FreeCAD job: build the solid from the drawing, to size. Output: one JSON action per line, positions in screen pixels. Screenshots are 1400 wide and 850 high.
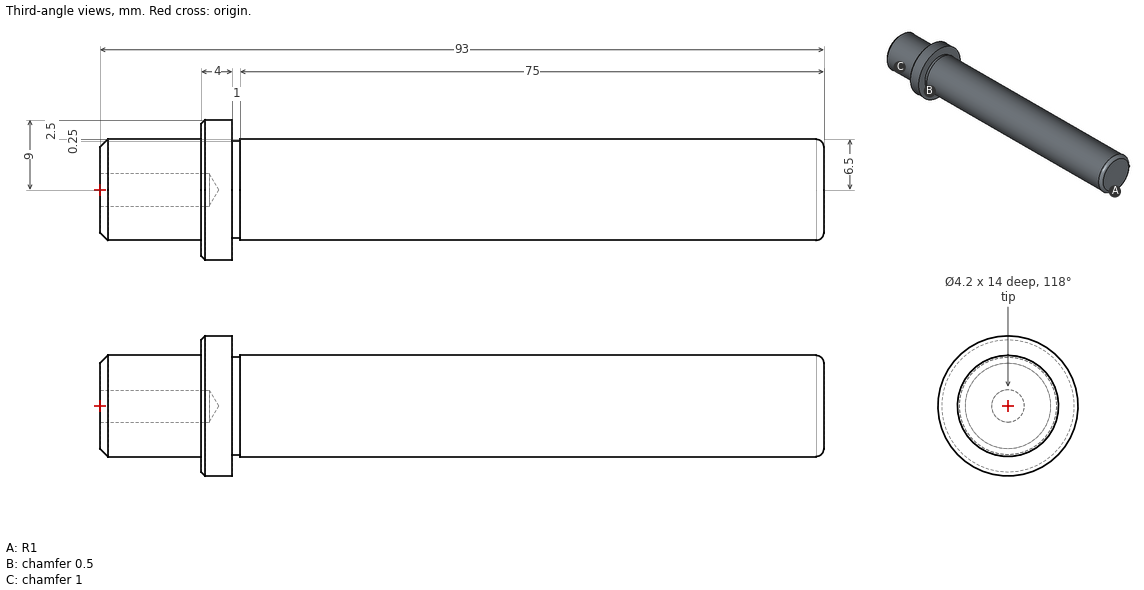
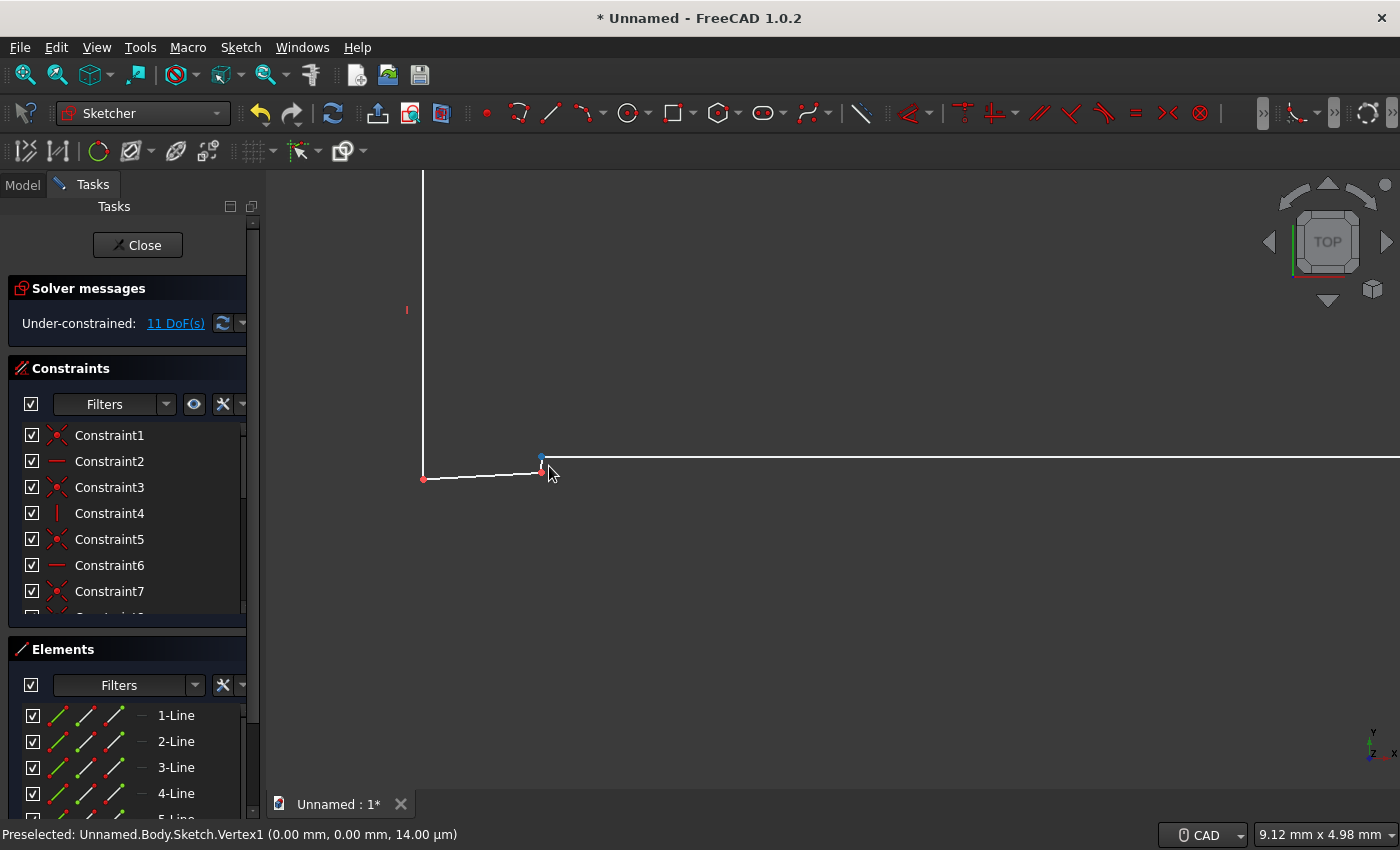
{"action": "left_click", "coordinate": [541, 465]}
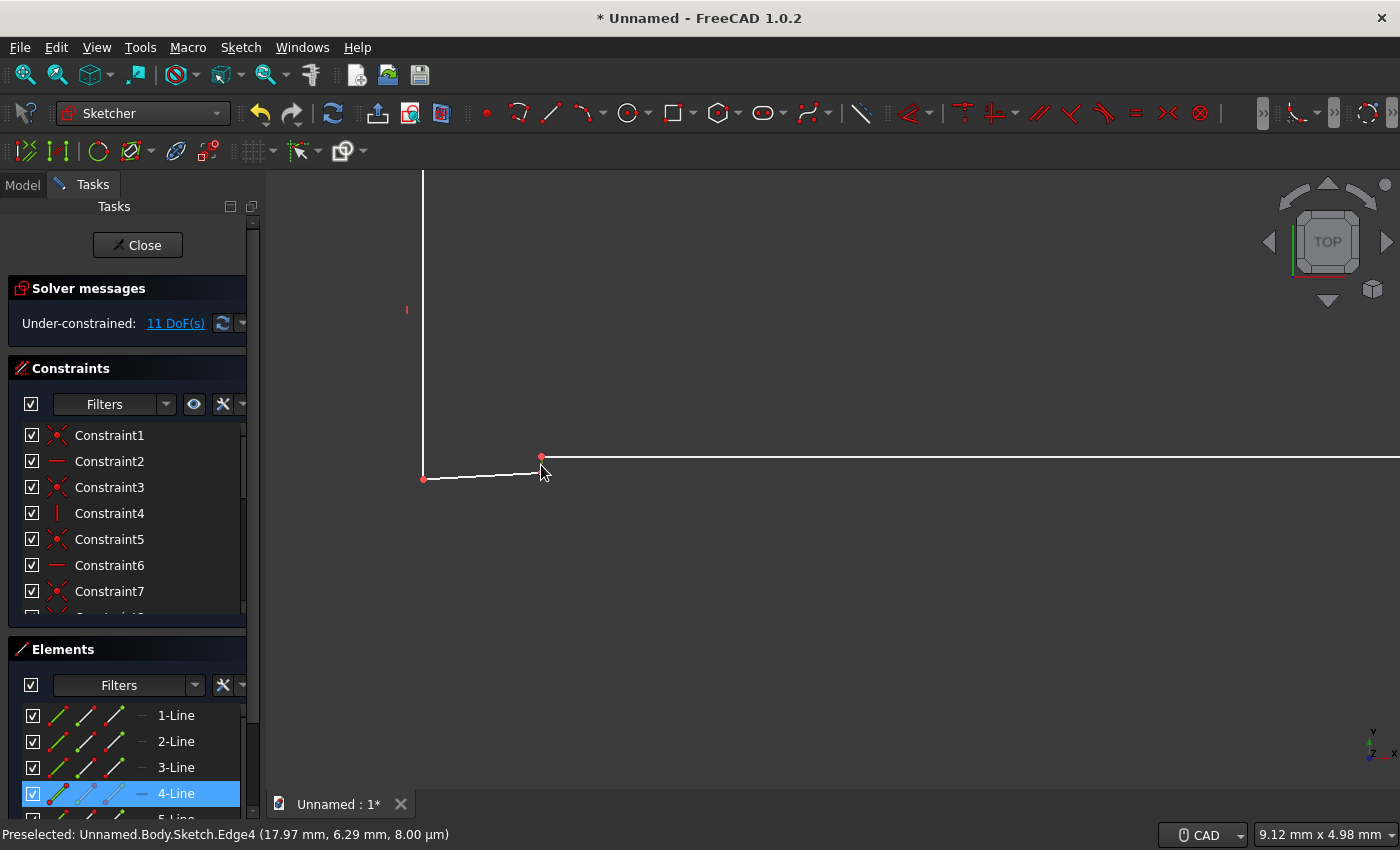
{"action": "key", "text": "v"}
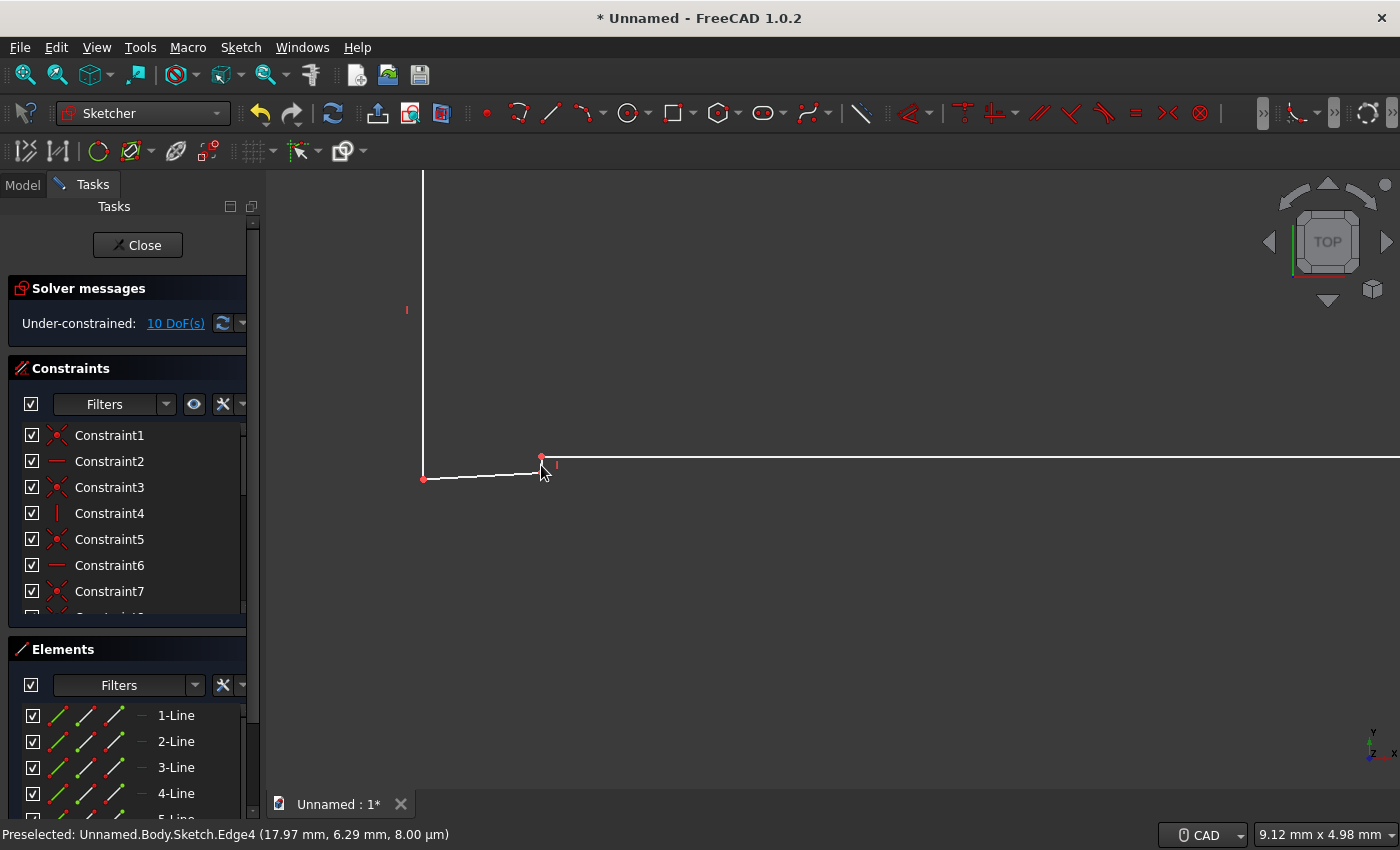
{"action": "left_click", "coordinate": [506, 475]}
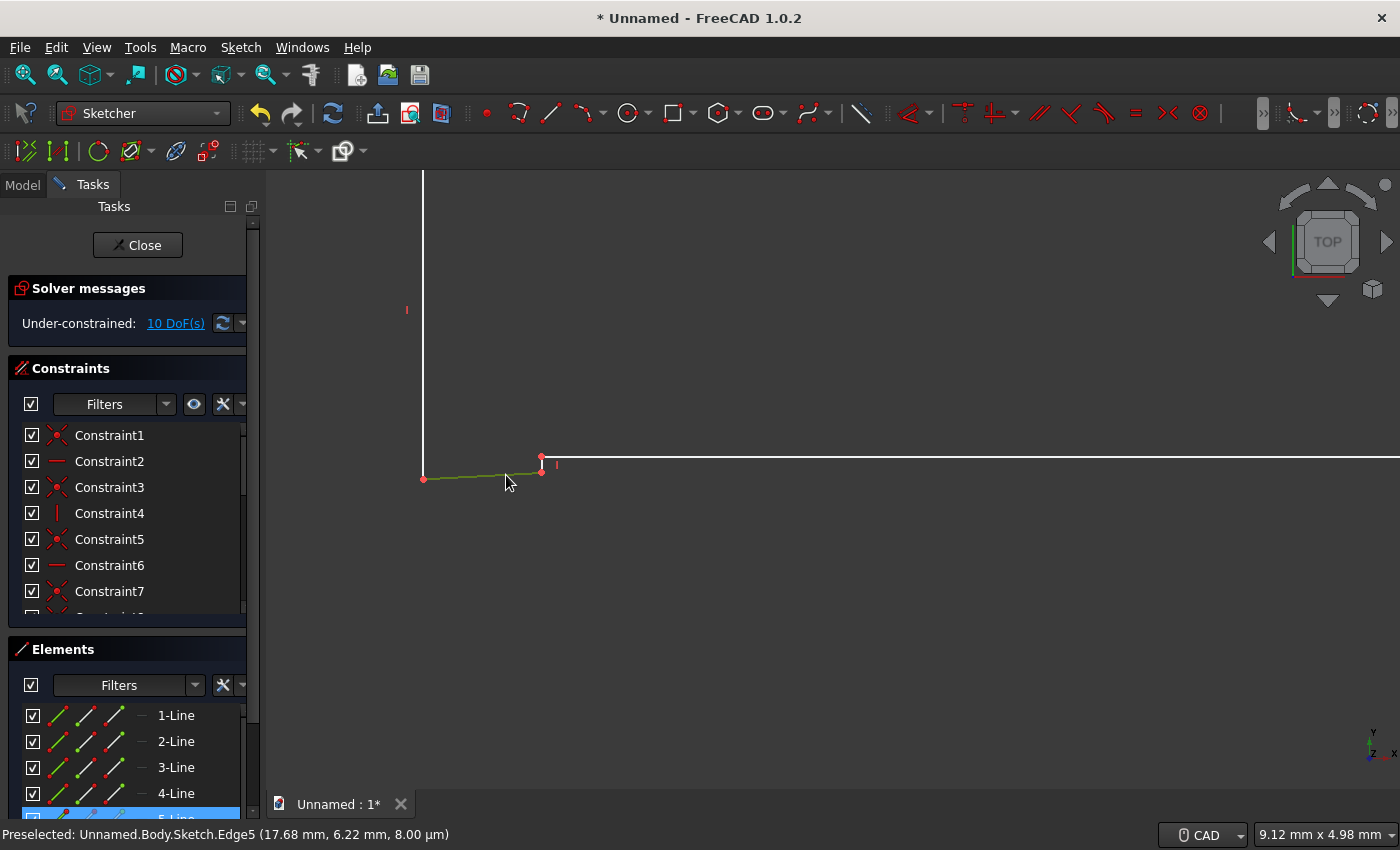
{"action": "key", "text": "h"}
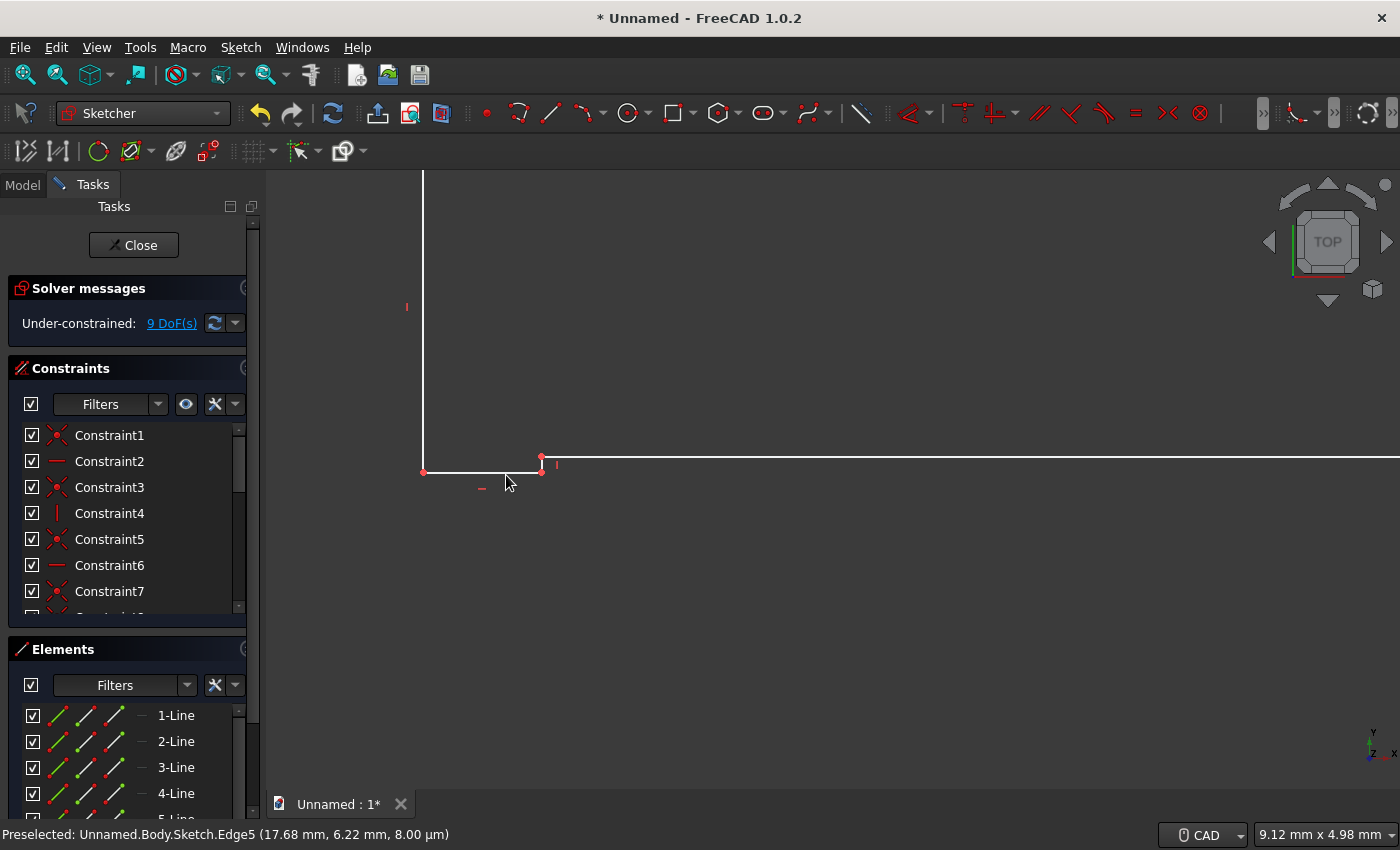
{"action": "scroll", "coordinate": [549, 466], "scroll_direction": "down", "scroll_amount": 14}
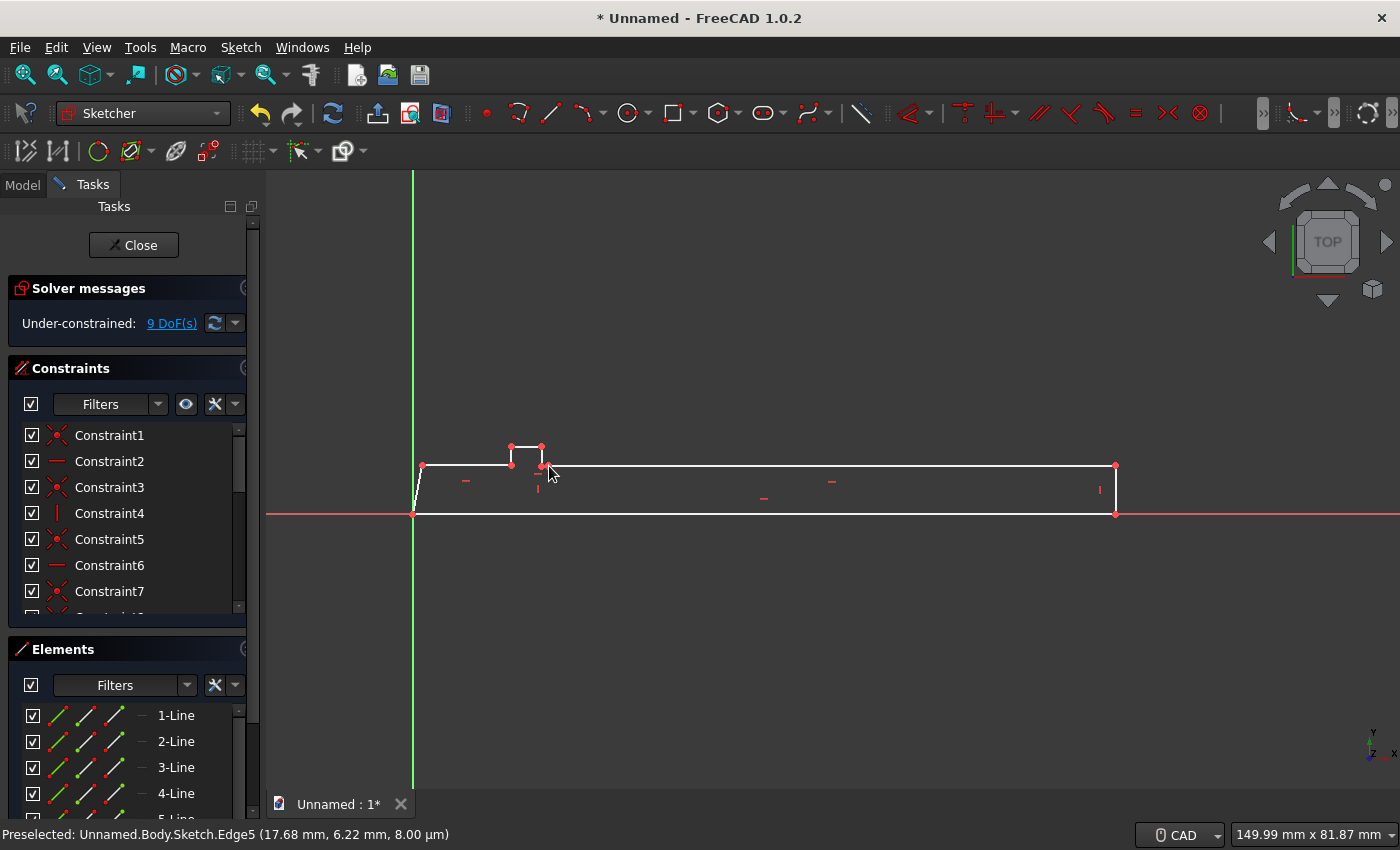
{"action": "scroll", "coordinate": [419, 480], "scroll_direction": "up", "scroll_amount": 4}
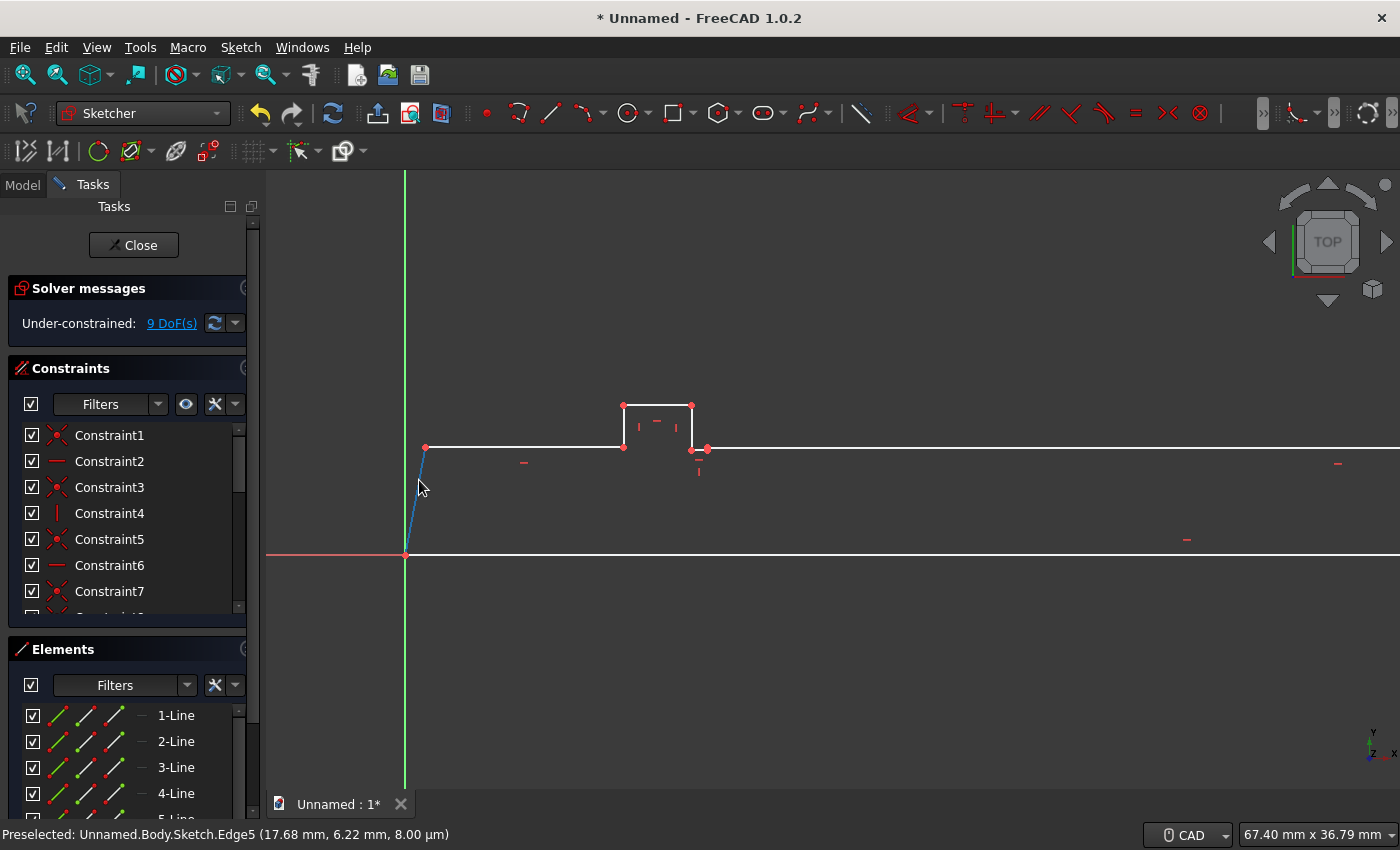
{"action": "left_click", "coordinate": [419, 479]}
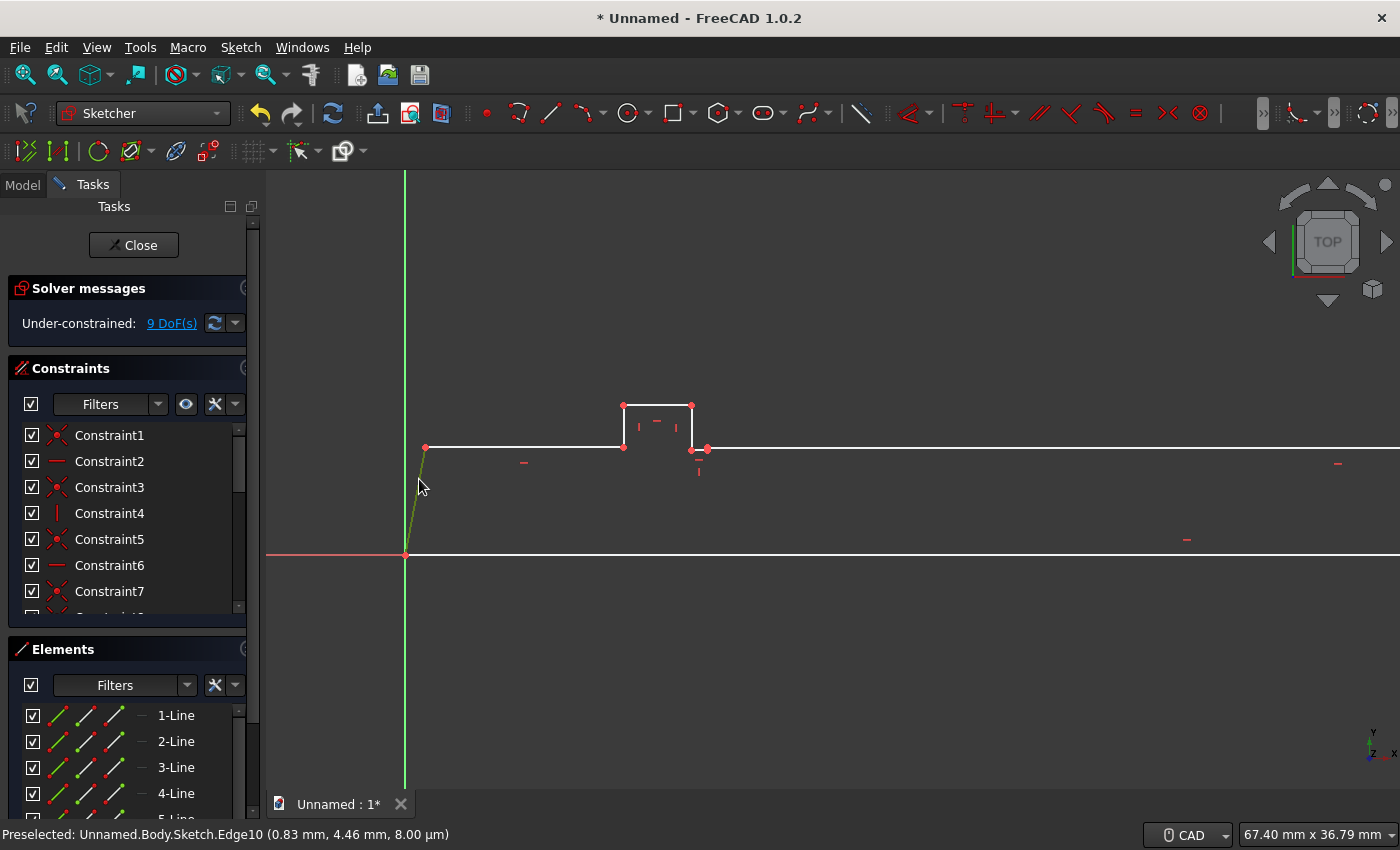
{"action": "key", "text": "v"}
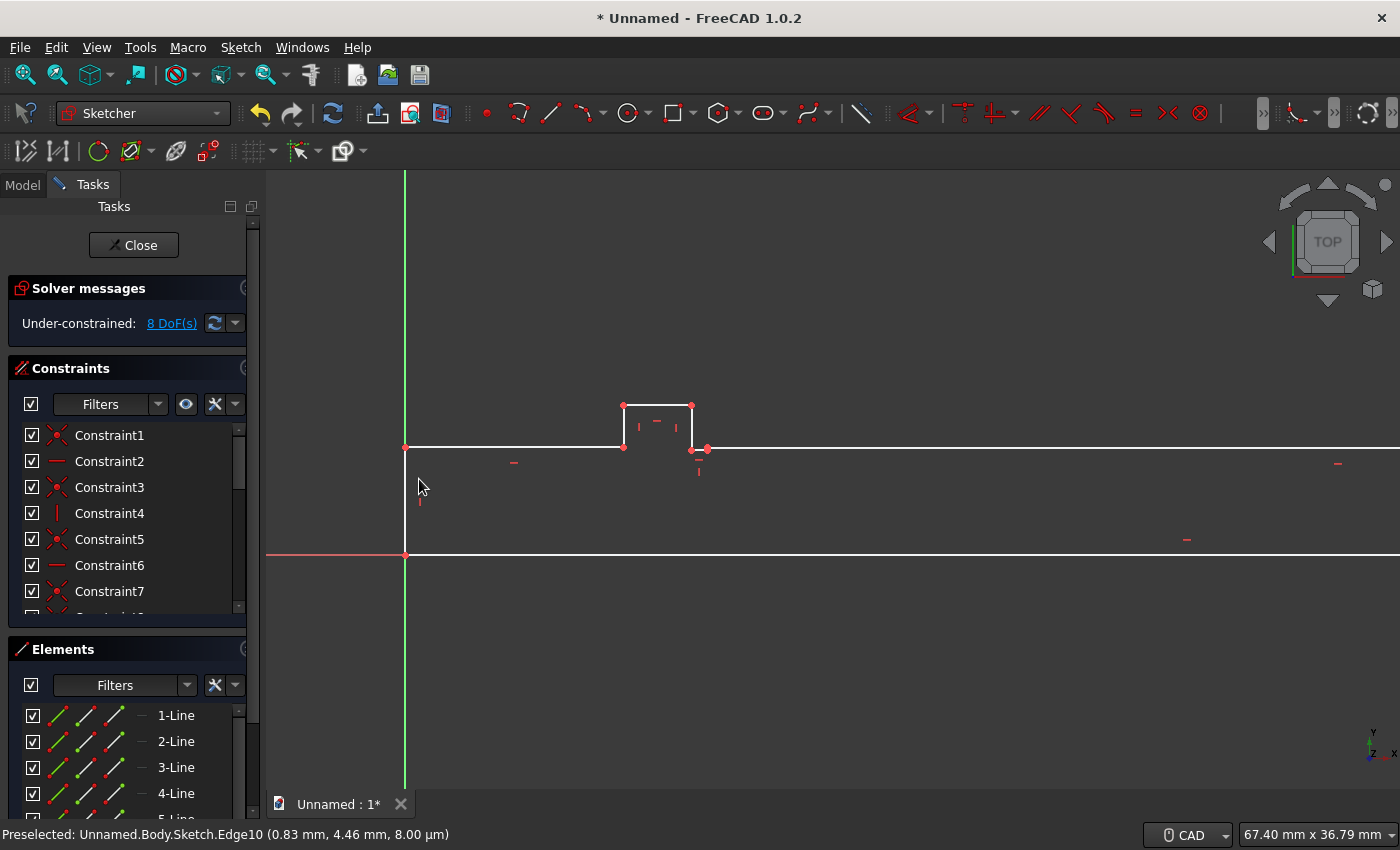
{"action": "key", "text": "d"}